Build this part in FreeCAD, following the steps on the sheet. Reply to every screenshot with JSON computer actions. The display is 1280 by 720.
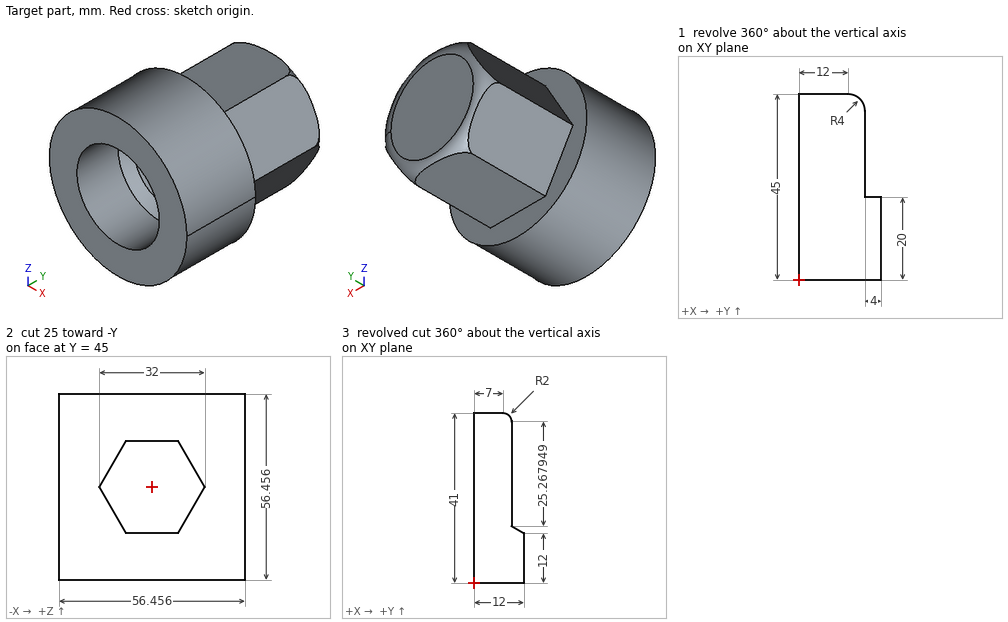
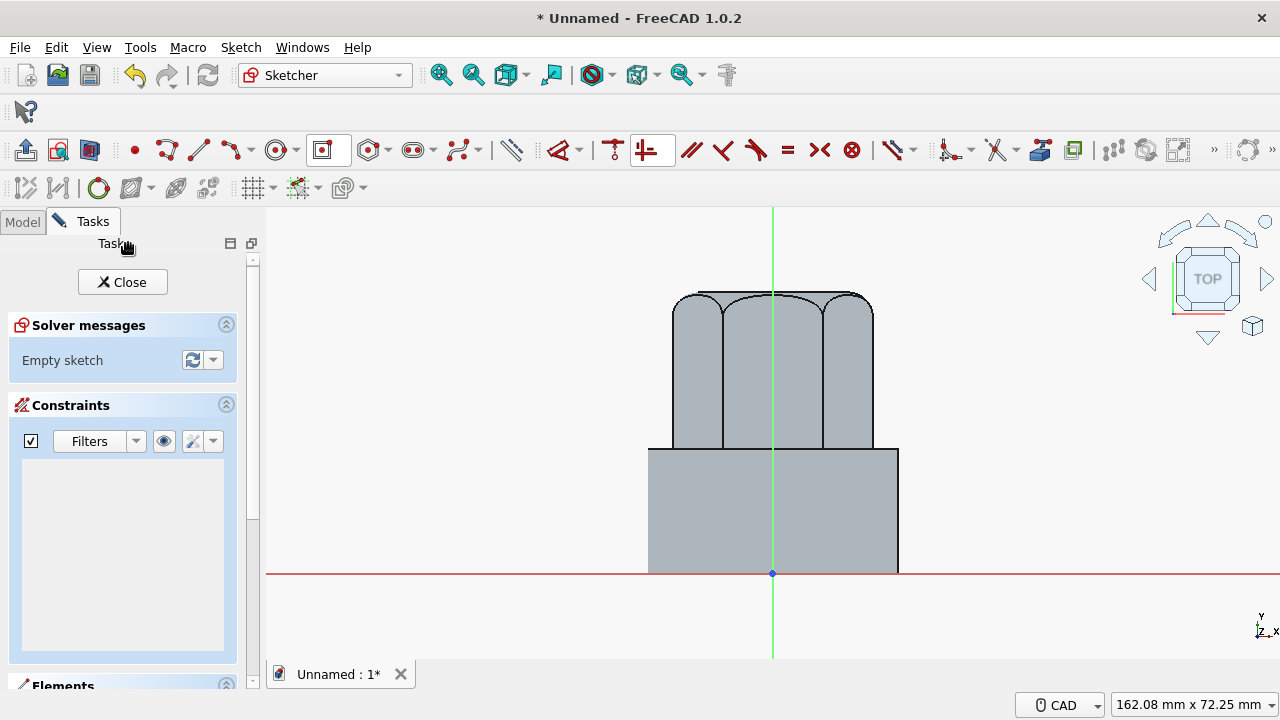
{"action": "left_click", "coordinate": [817, 317]}
{"action": "left_click", "coordinate": [773, 317]}
{"action": "left_click", "coordinate": [773, 574]}
{"action": "left_click", "coordinate": [848, 565]}
{"action": "left_click", "coordinate": [848, 499]}
{"action": "left_click", "coordinate": [829, 488]}
{"action": "left_click", "coordinate": [829, 330]}
{"action": "right_click", "coordinate": [829, 330]}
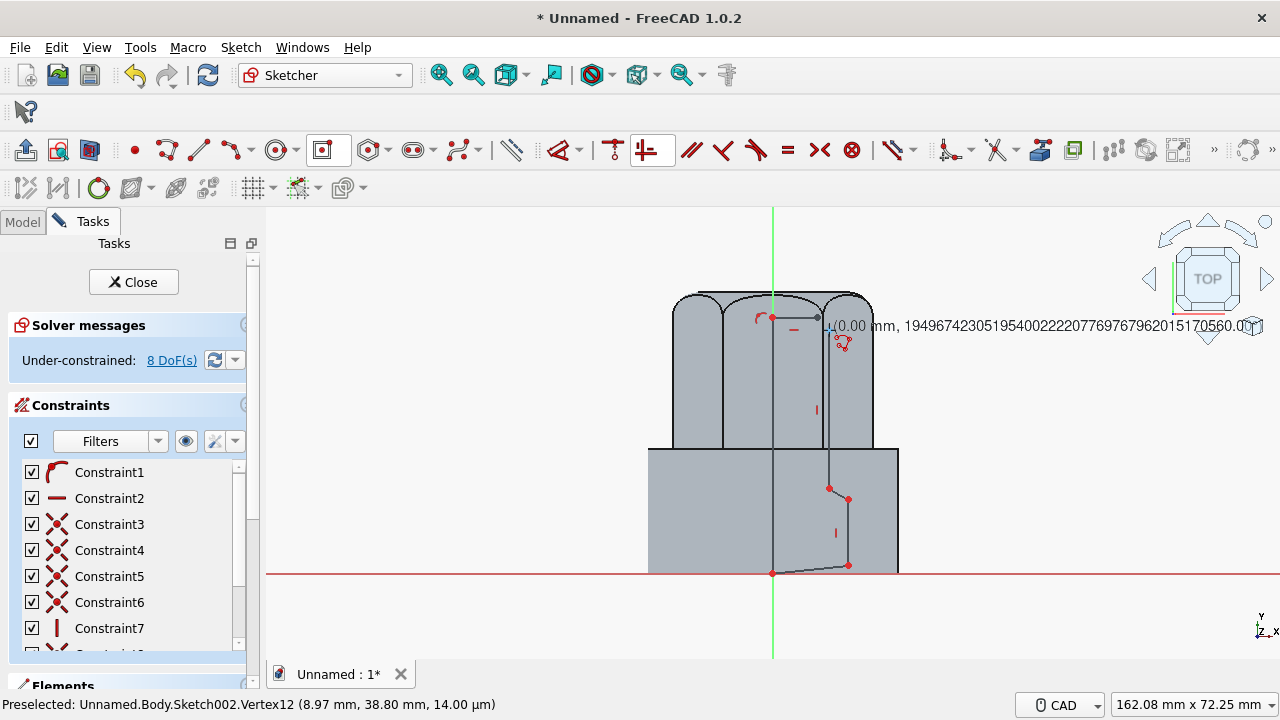
{"action": "key", "text": "g 3 a"}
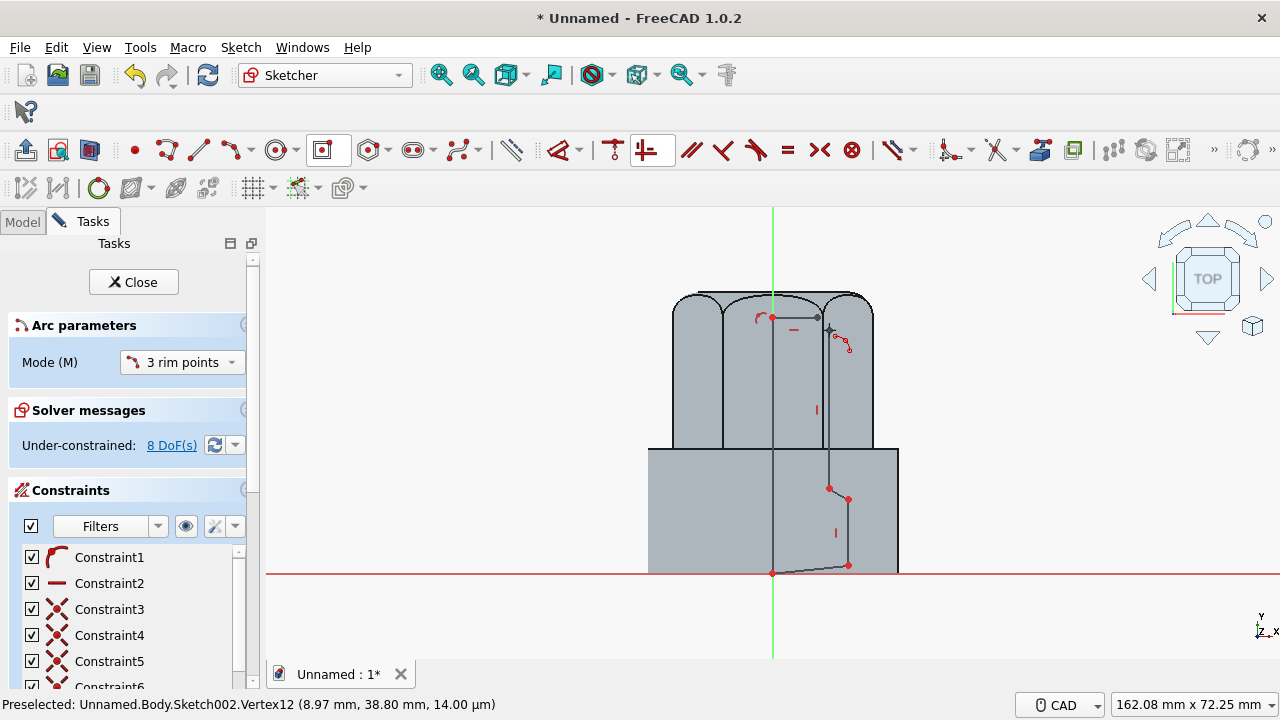
{"action": "left_click", "coordinate": [829, 331]}
{"action": "left_click", "coordinate": [817, 318]}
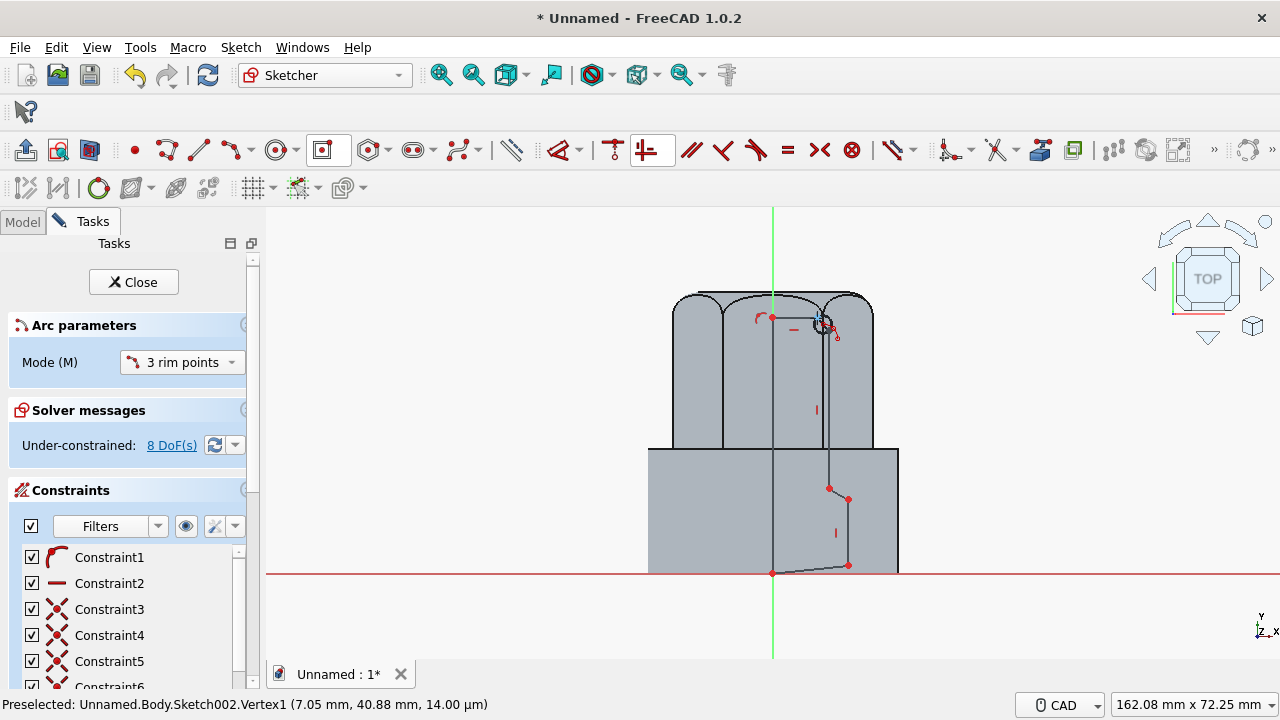
{"action": "scroll", "coordinate": [826, 321], "scroll_direction": "up", "scroll_amount": 8}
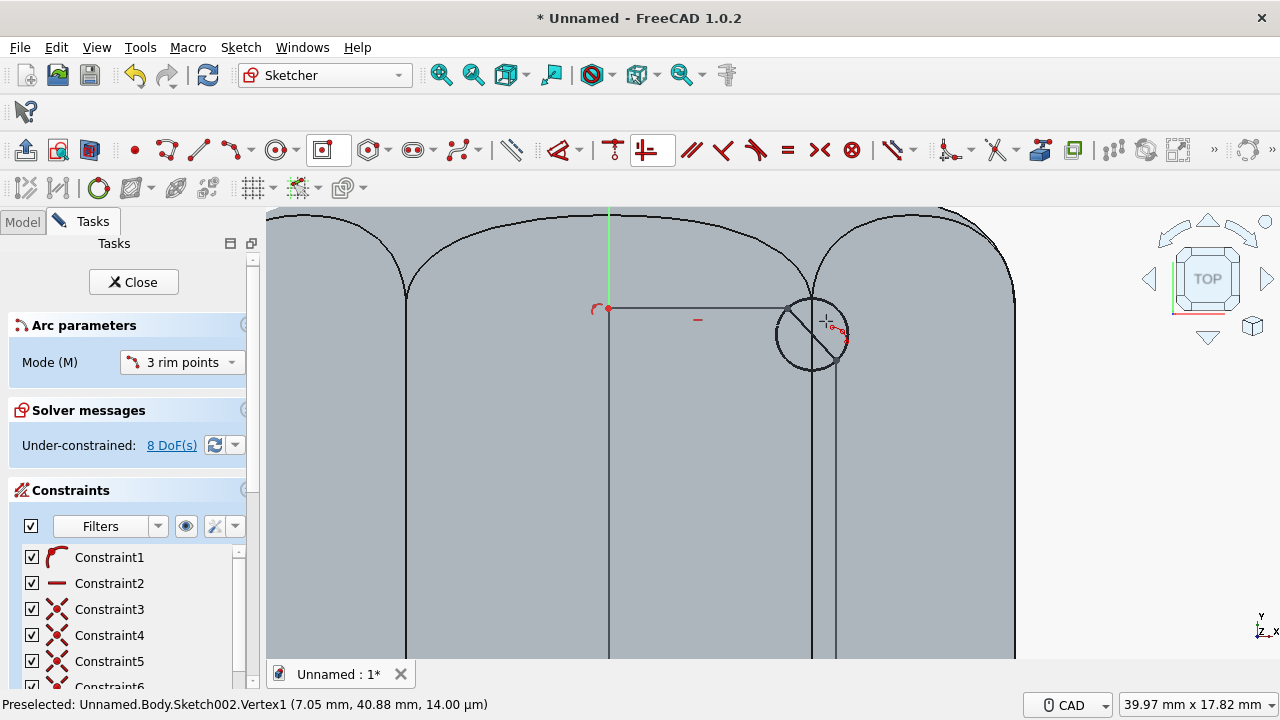
{"action": "left_click", "coordinate": [821, 320]}
{"action": "key", "text": "Escape"}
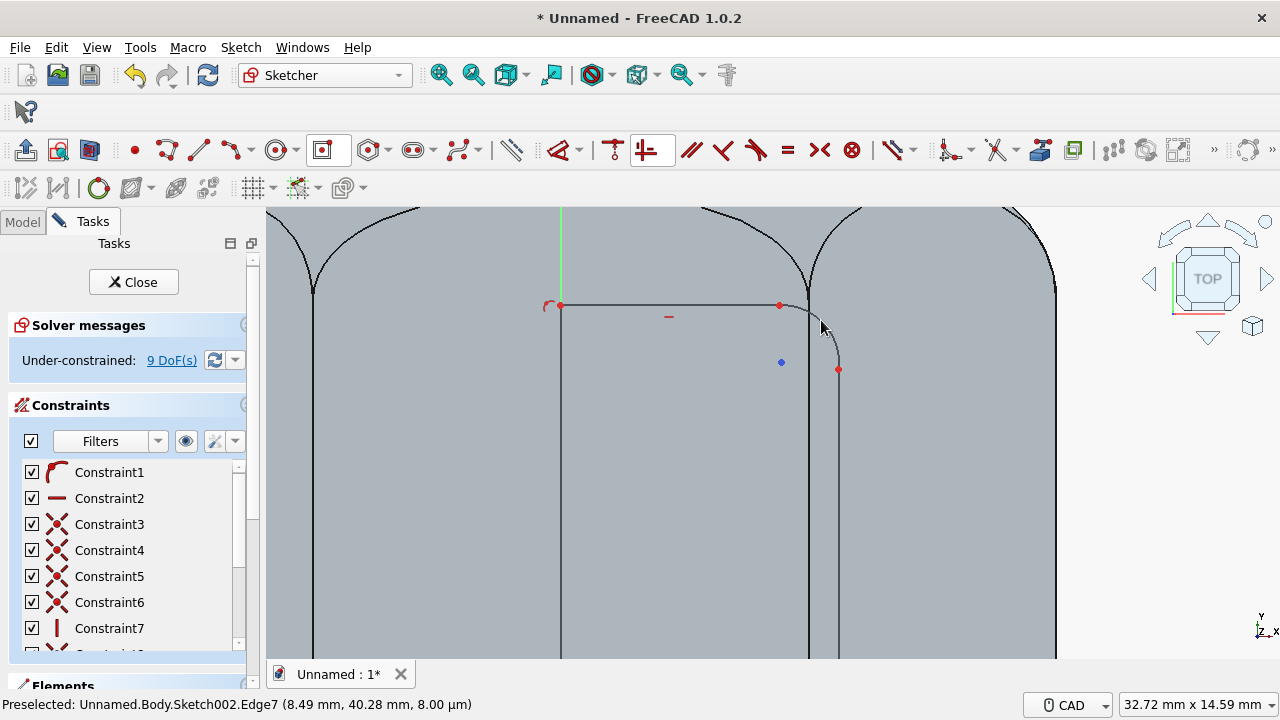
{"action": "scroll", "coordinate": [694, 306], "scroll_direction": "down", "scroll_amount": 8}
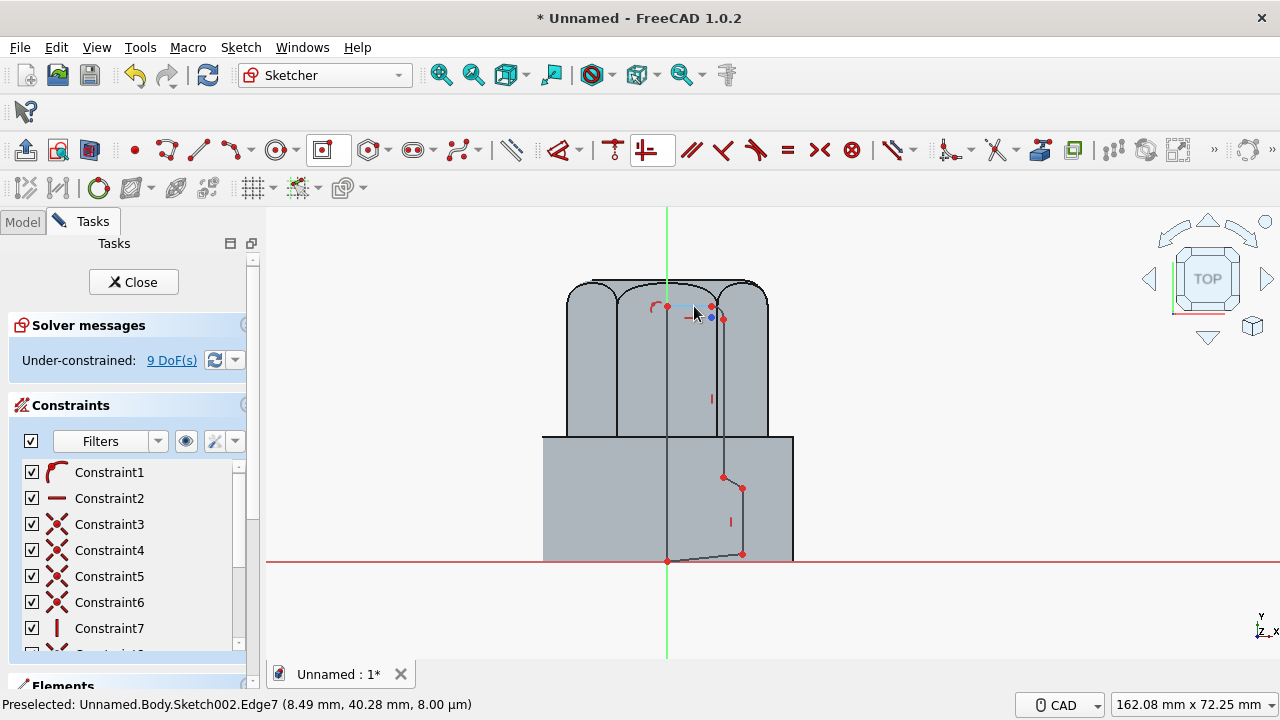
{"action": "left_click", "coordinate": [698, 306]}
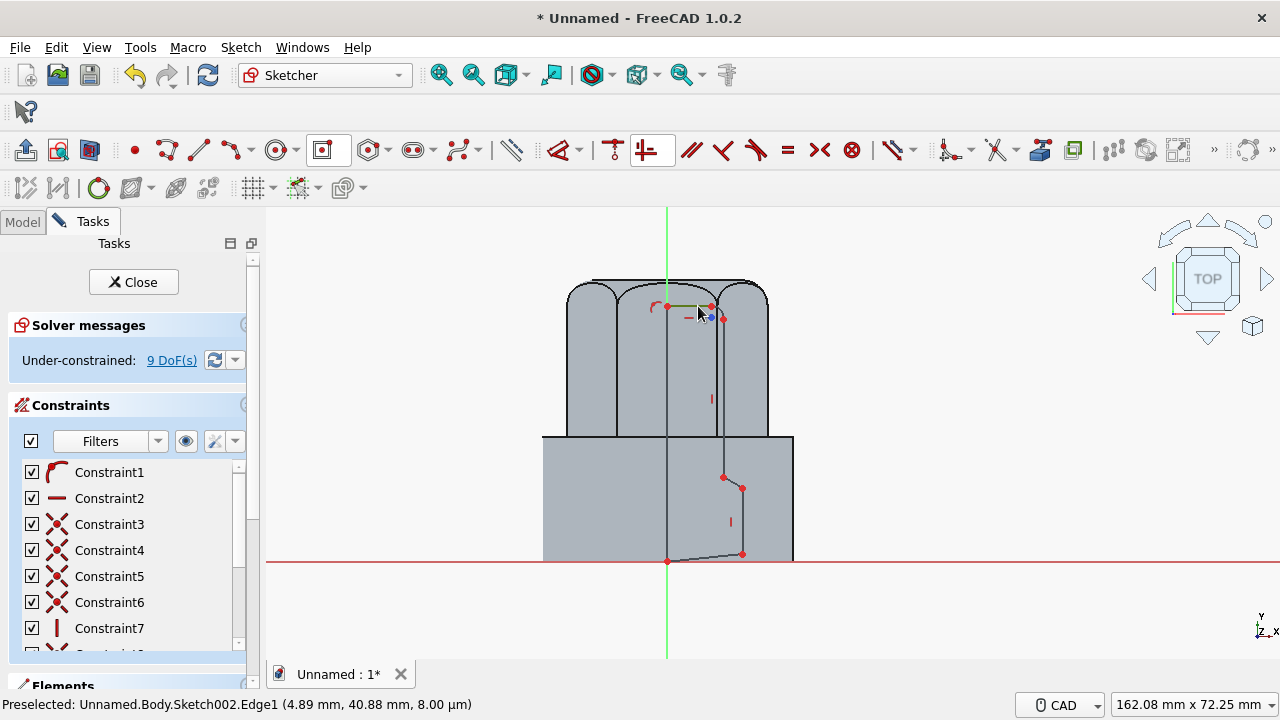
{"action": "scroll", "coordinate": [721, 310], "scroll_direction": "up", "scroll_amount": 2}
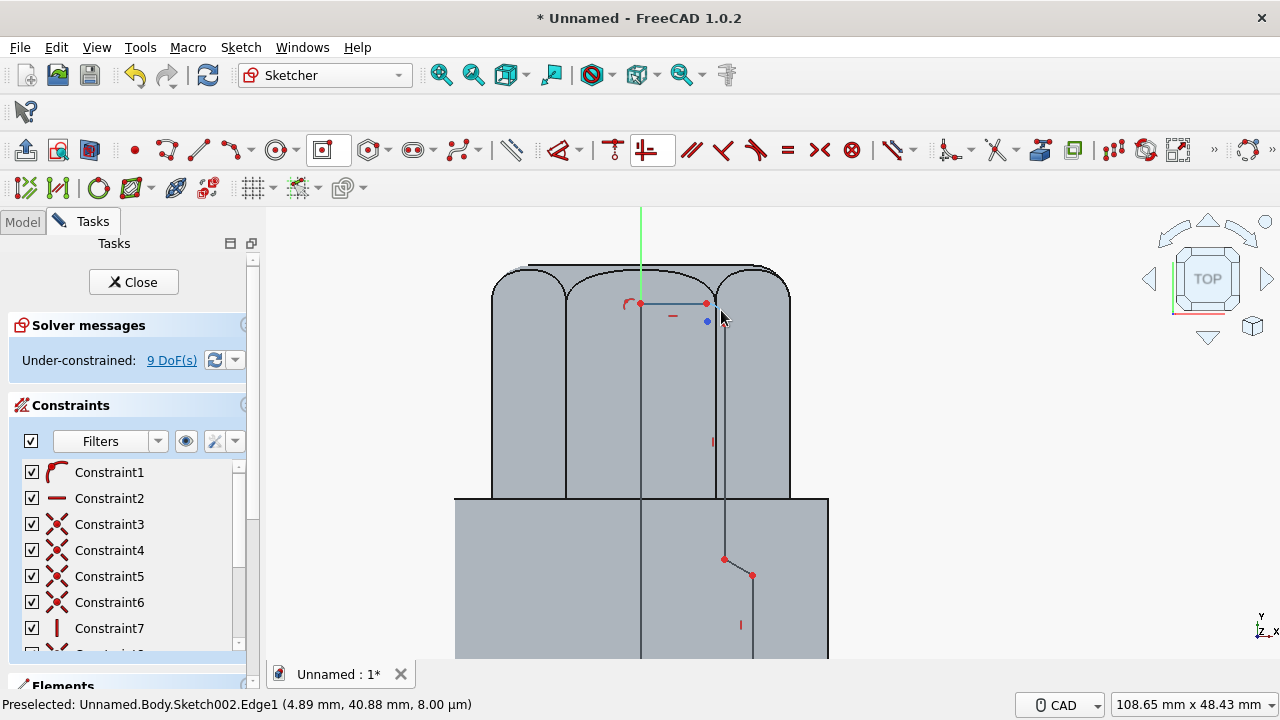
{"action": "left_click", "coordinate": [720, 310]}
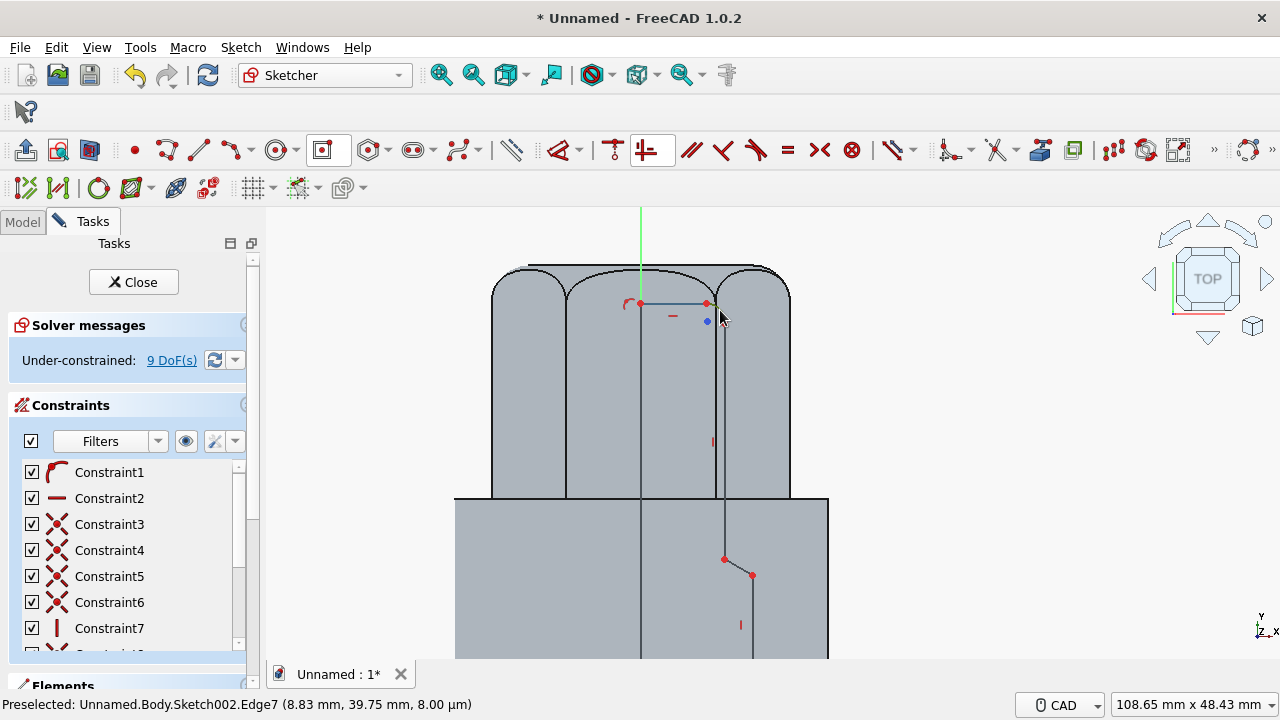
{"action": "key", "text": "t"}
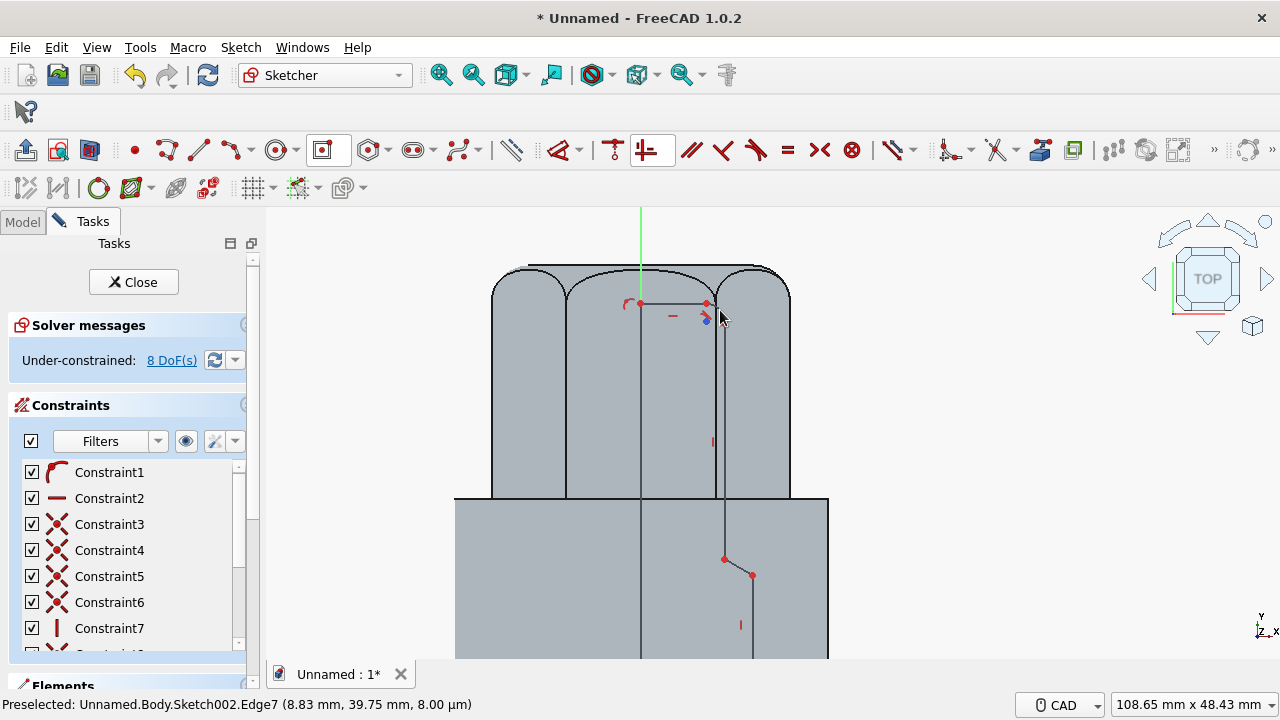
{"action": "left_click", "coordinate": [725, 488]}